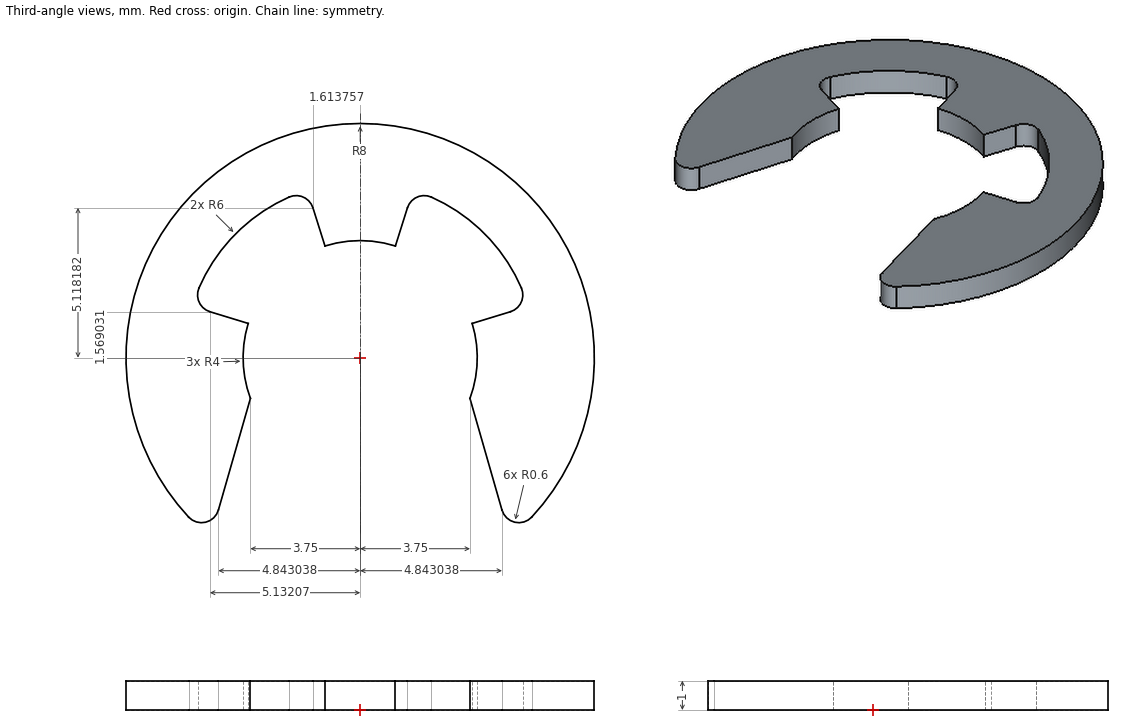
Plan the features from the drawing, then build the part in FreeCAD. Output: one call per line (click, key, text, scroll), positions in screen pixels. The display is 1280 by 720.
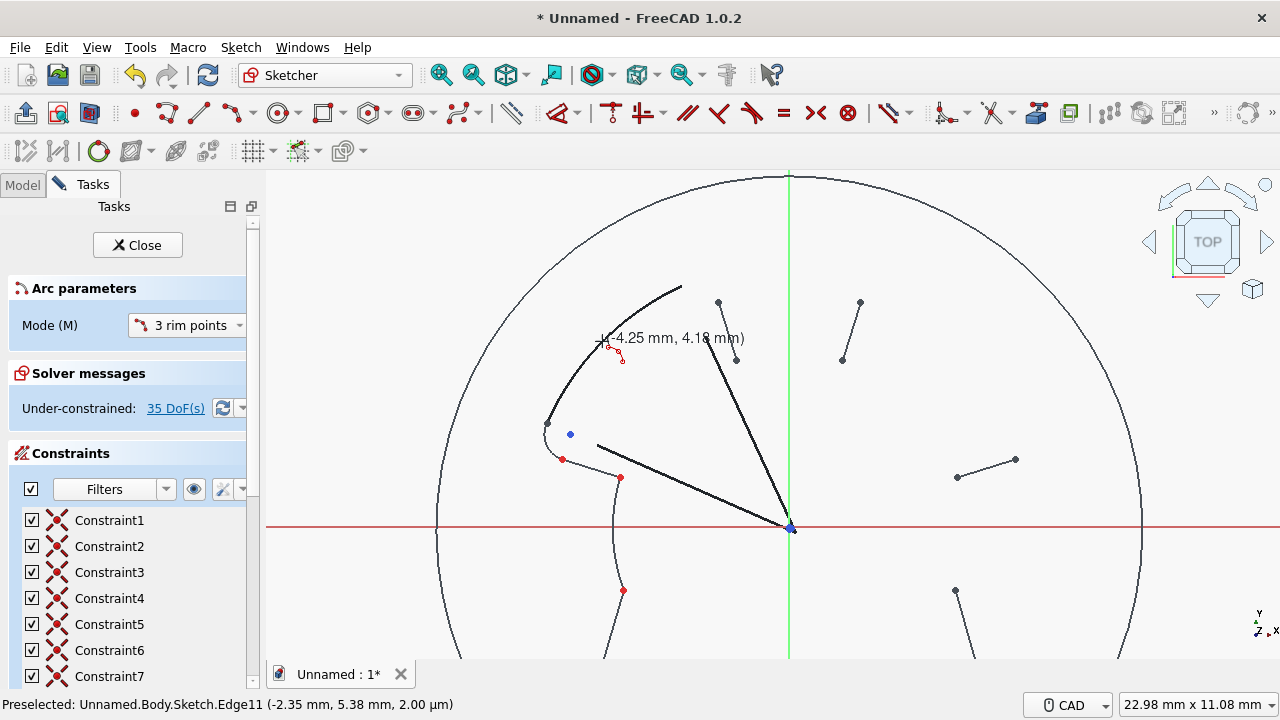
click(601, 341)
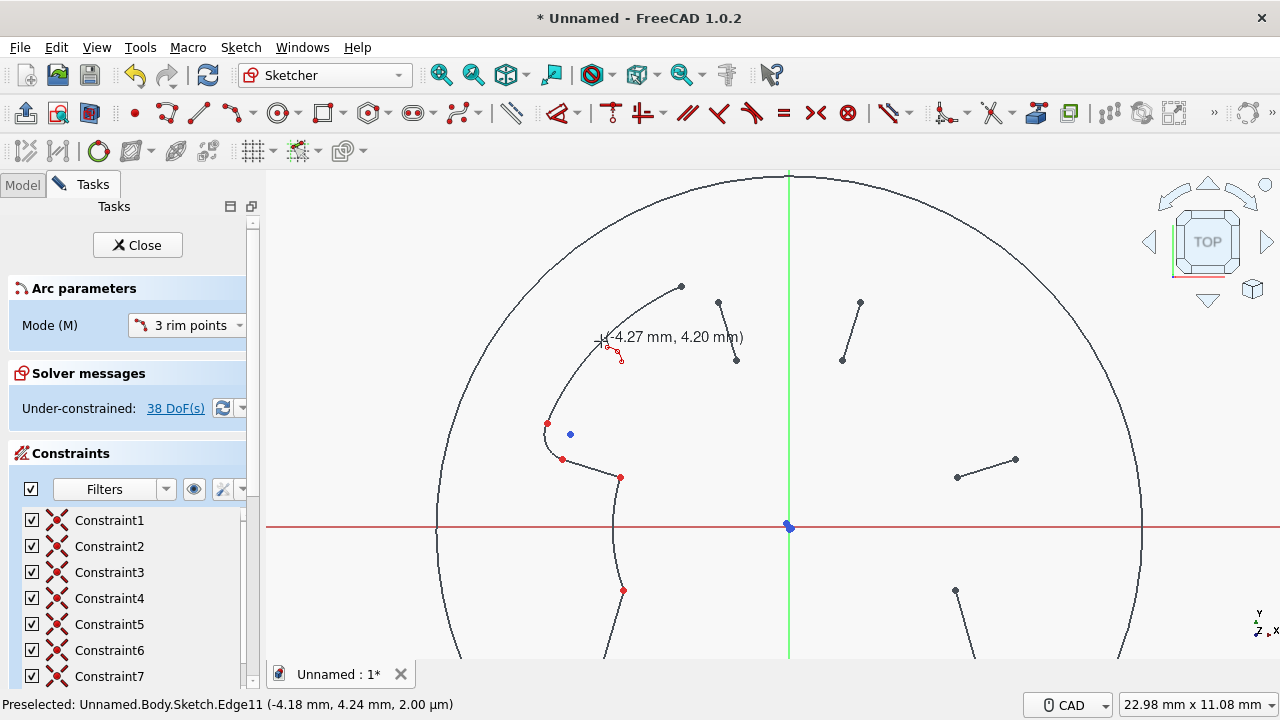
click(682, 286)
click(719, 303)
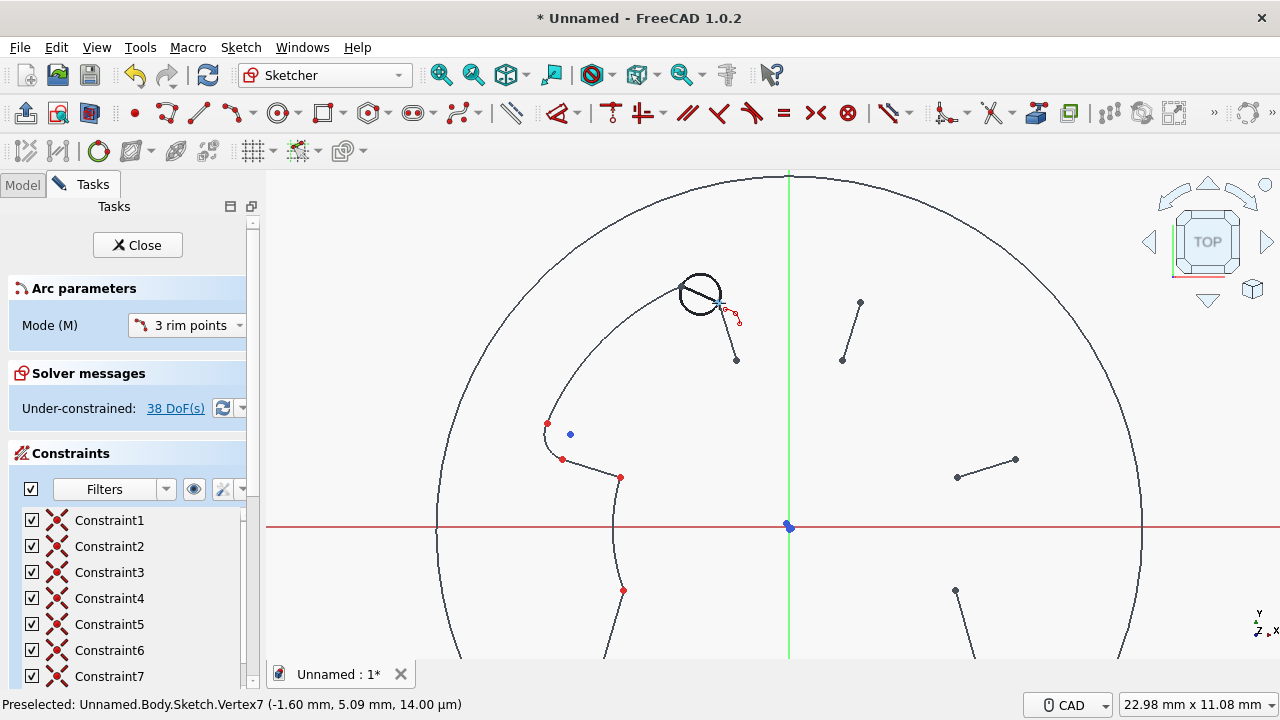
scroll(704, 285, up, 3)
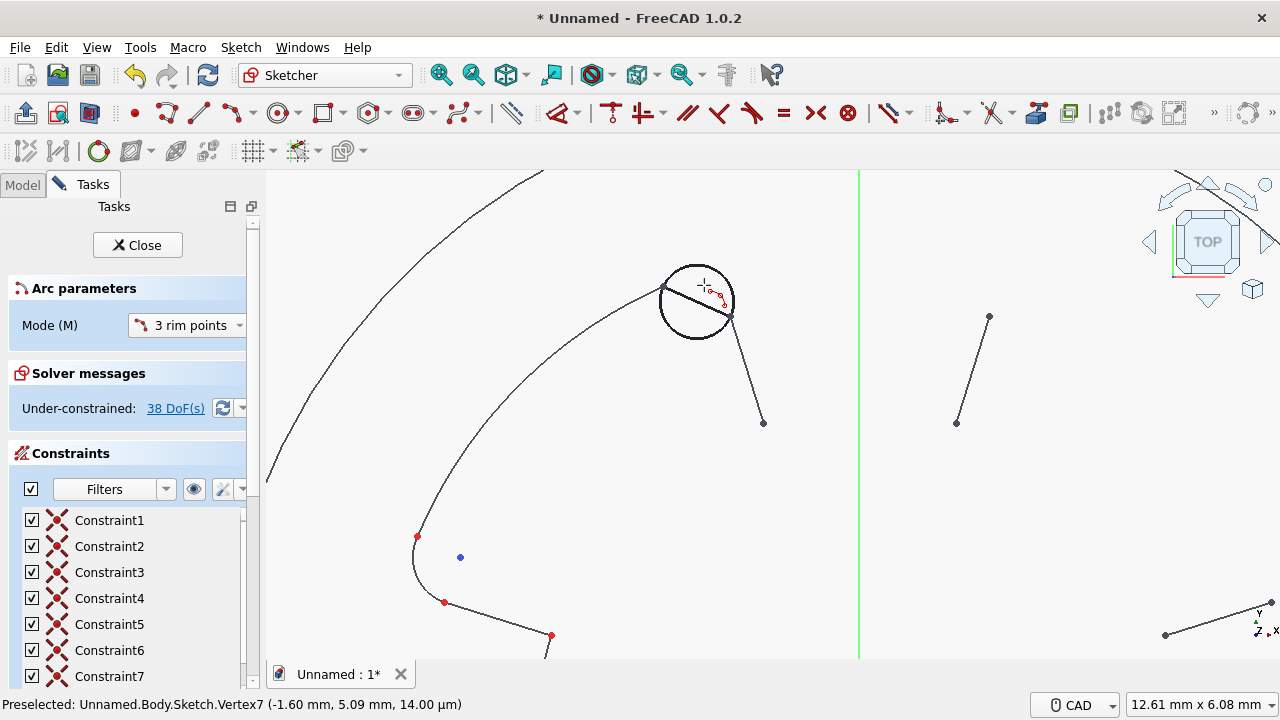
click(703, 285)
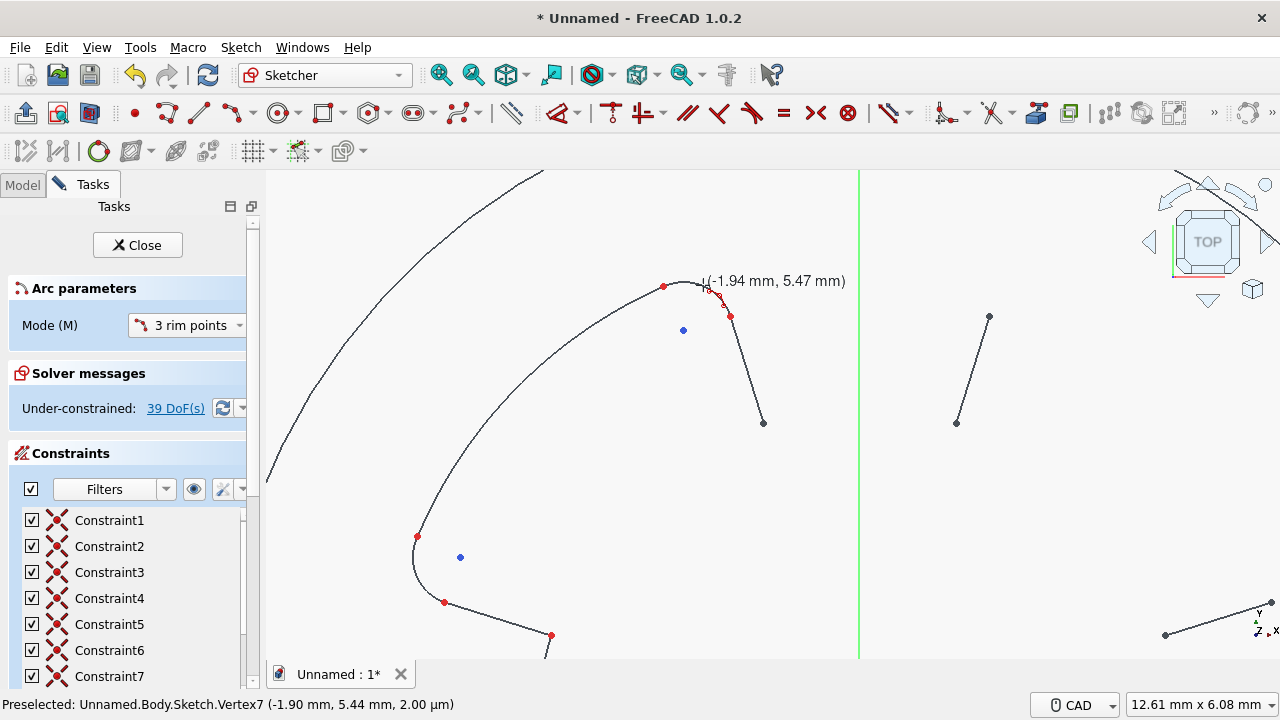
click(764, 423)
click(956, 423)
click(879, 405)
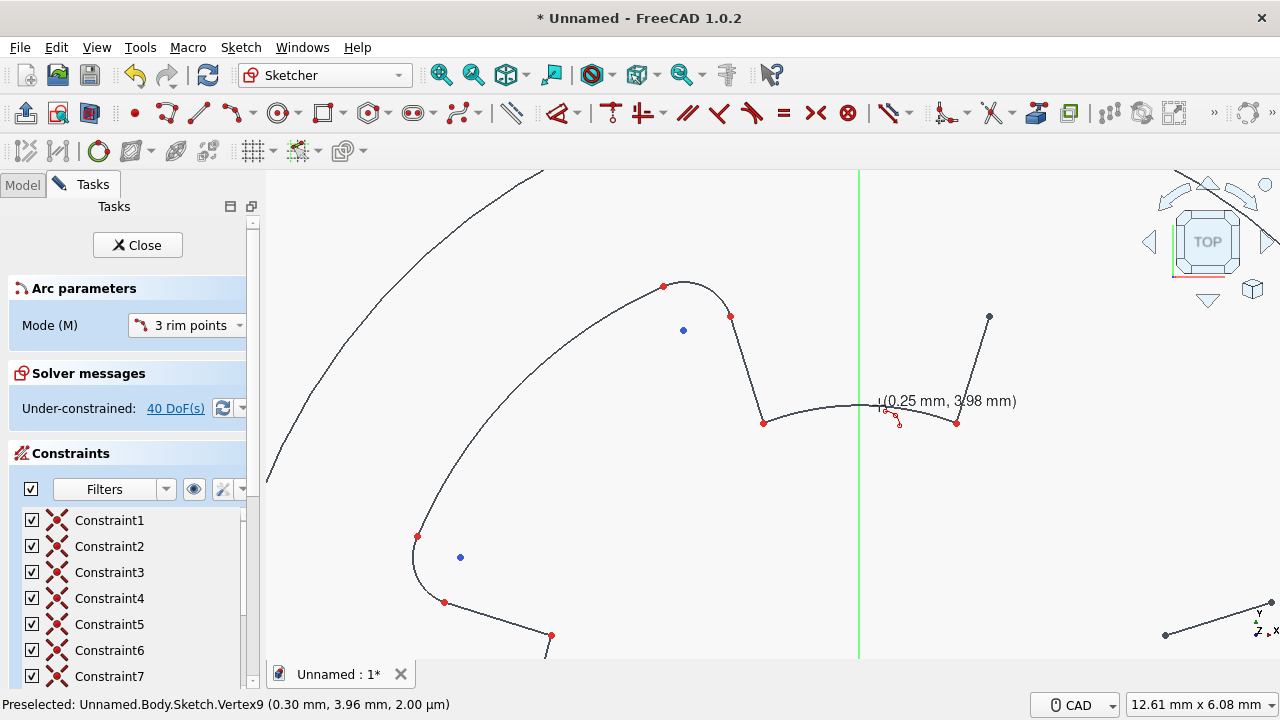
click(989, 317)
click(1054, 285)
click(1015, 285)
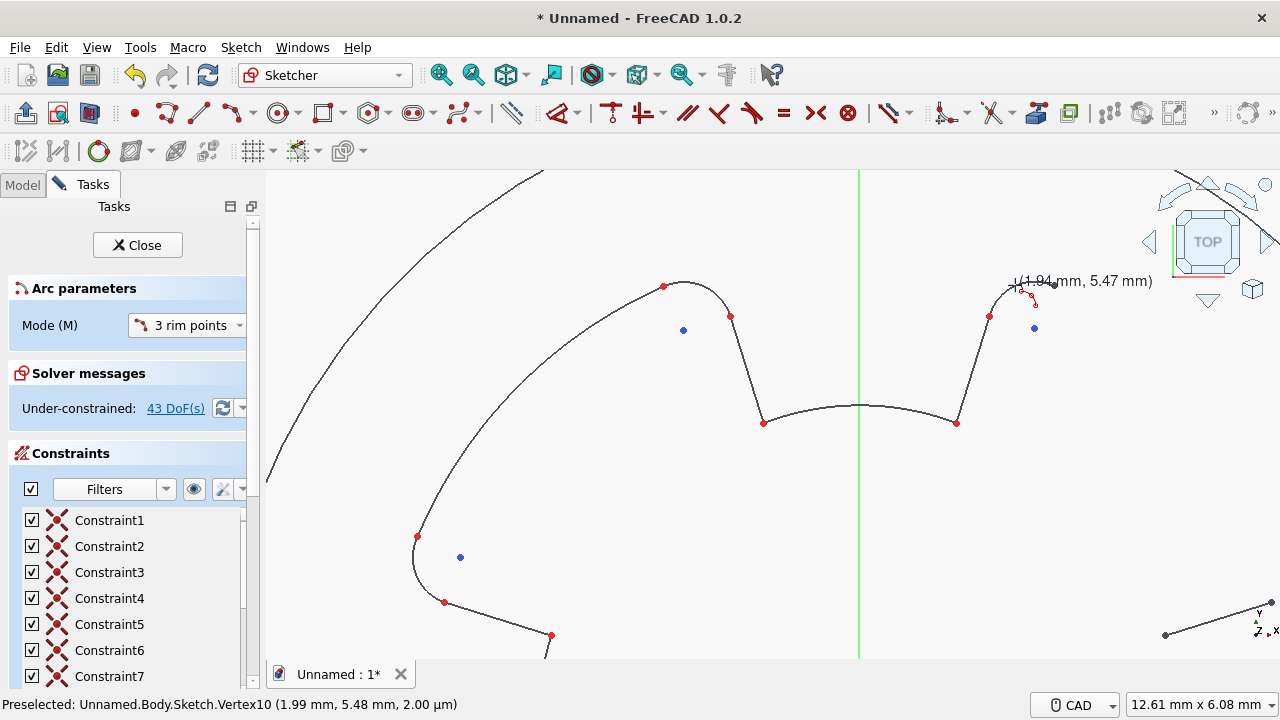
click(1054, 286)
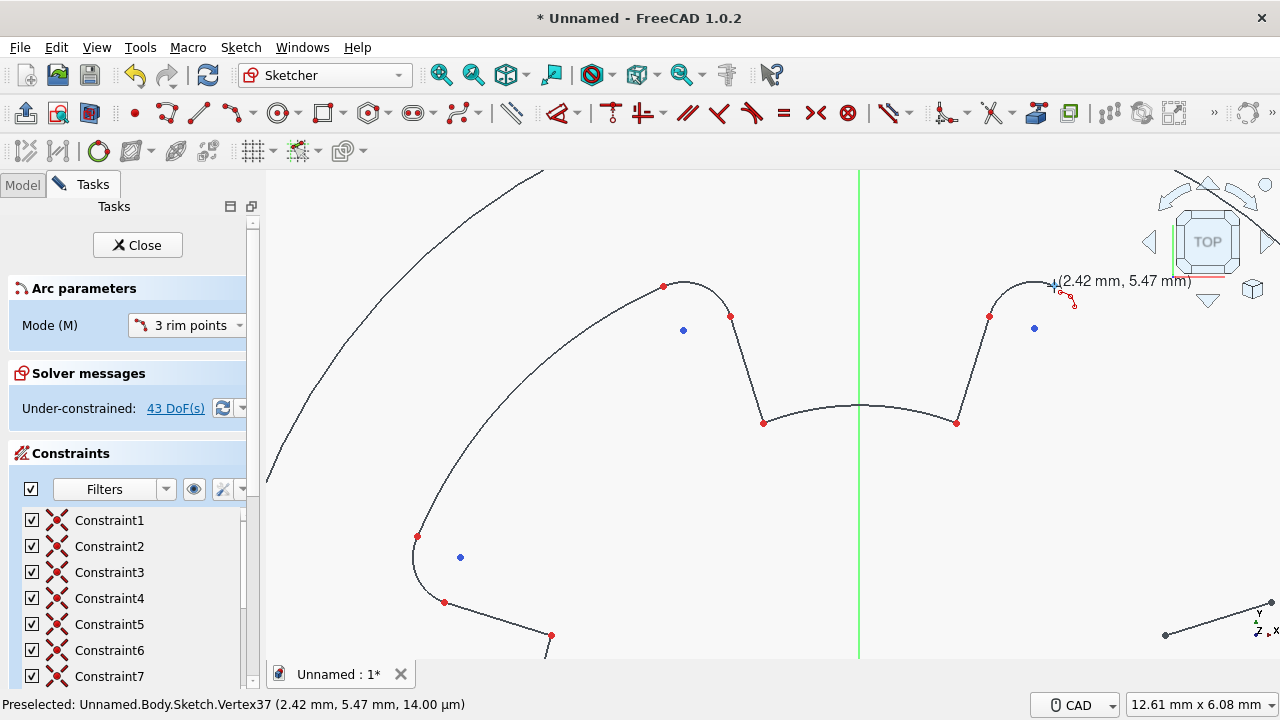
scroll(638, 321, down, 6)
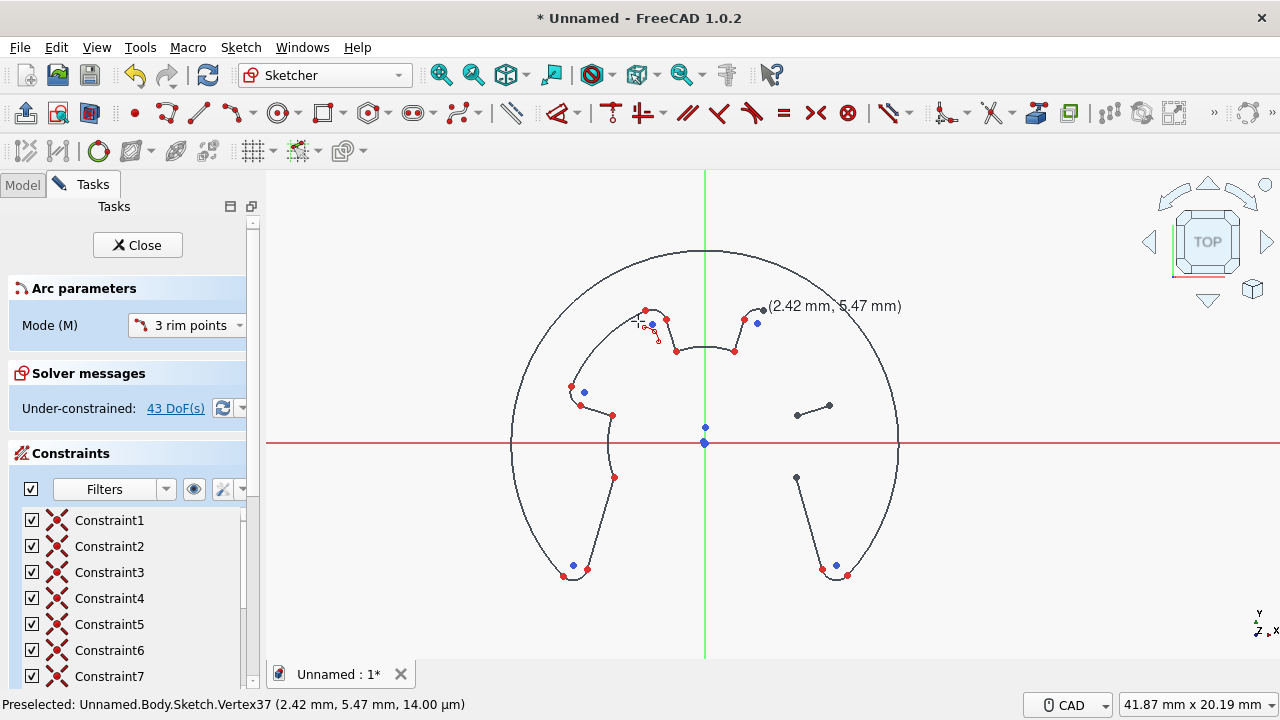
click(838, 386)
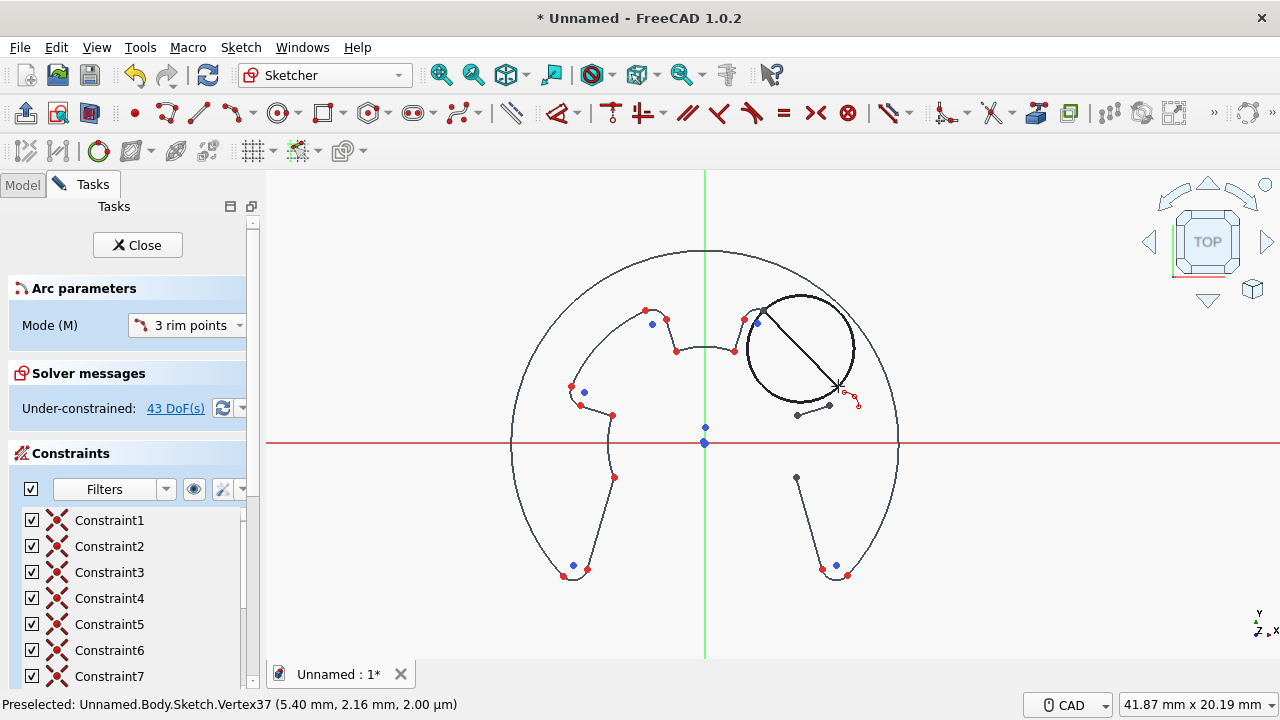
scroll(808, 341, up, 3)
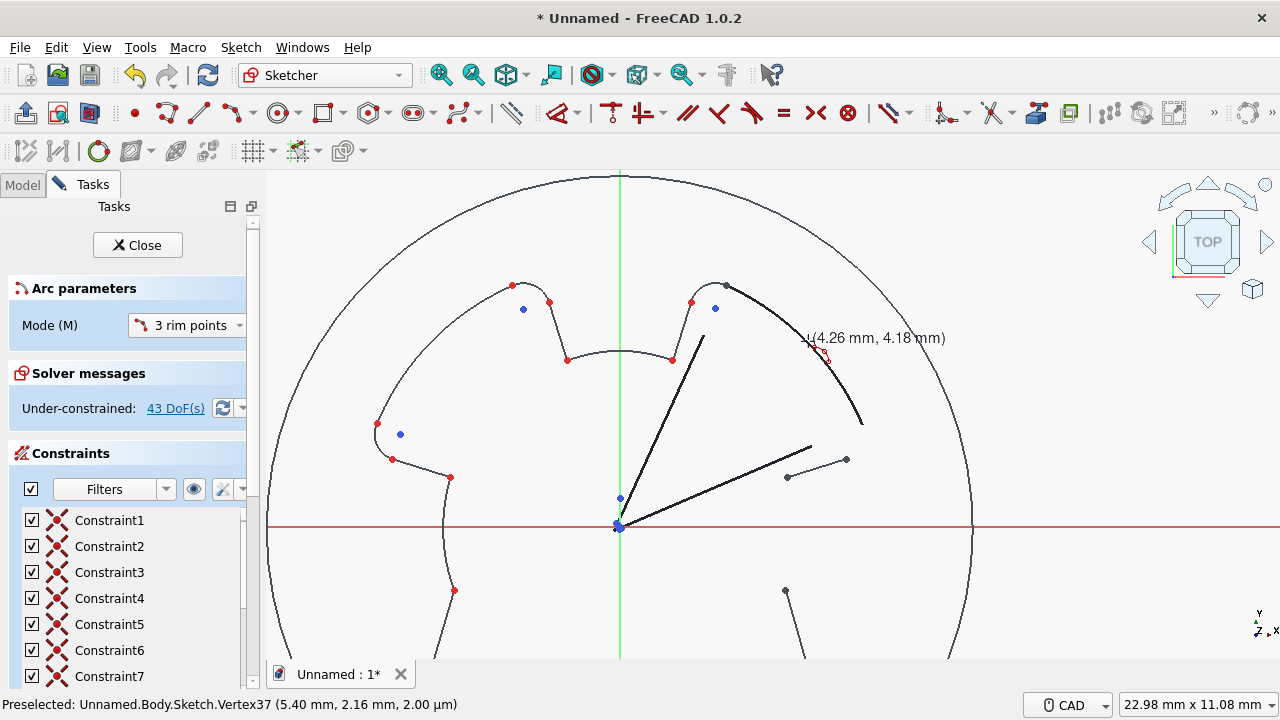
click(808, 341)